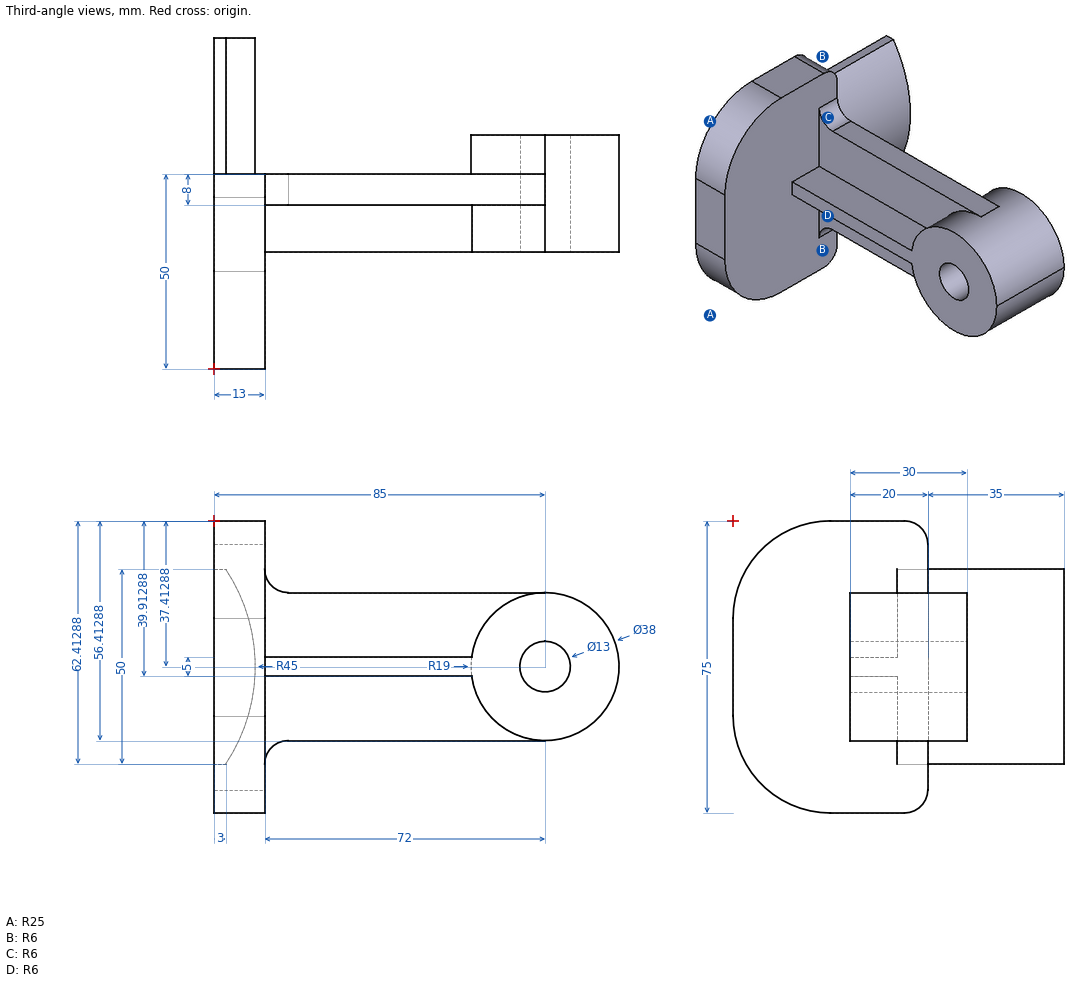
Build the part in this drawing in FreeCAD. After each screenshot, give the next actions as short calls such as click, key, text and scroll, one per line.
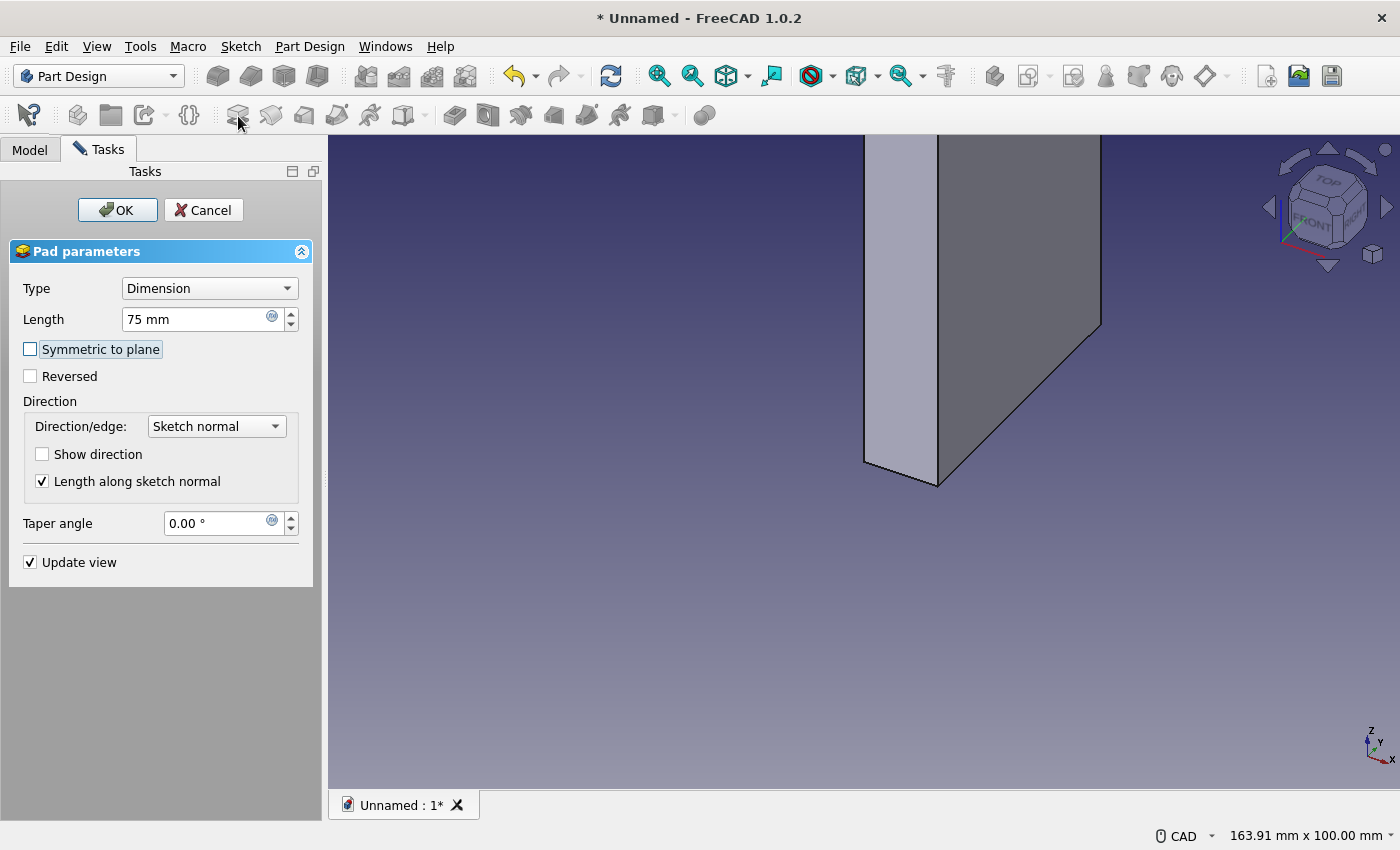
click(31, 376)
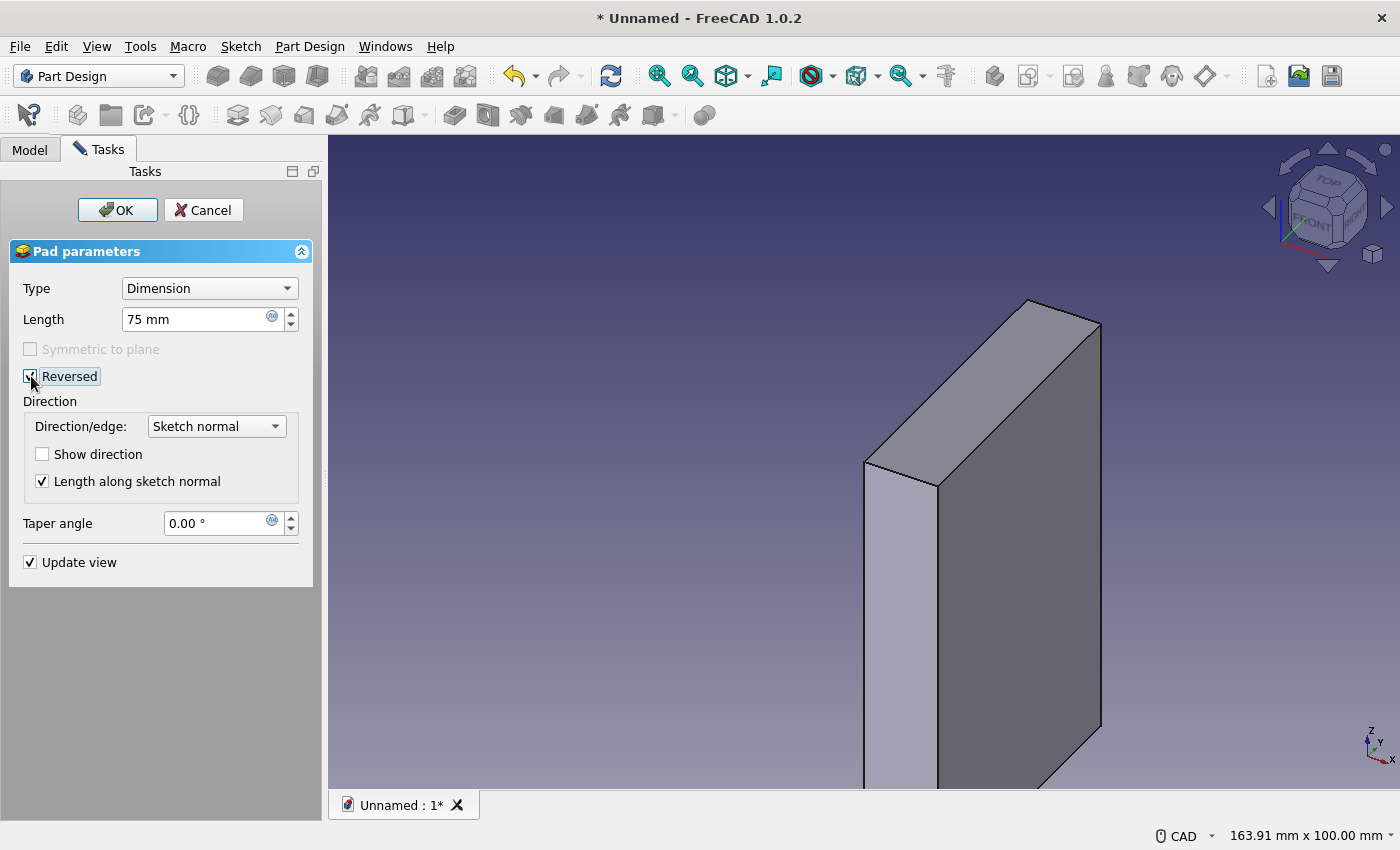
click(118, 210)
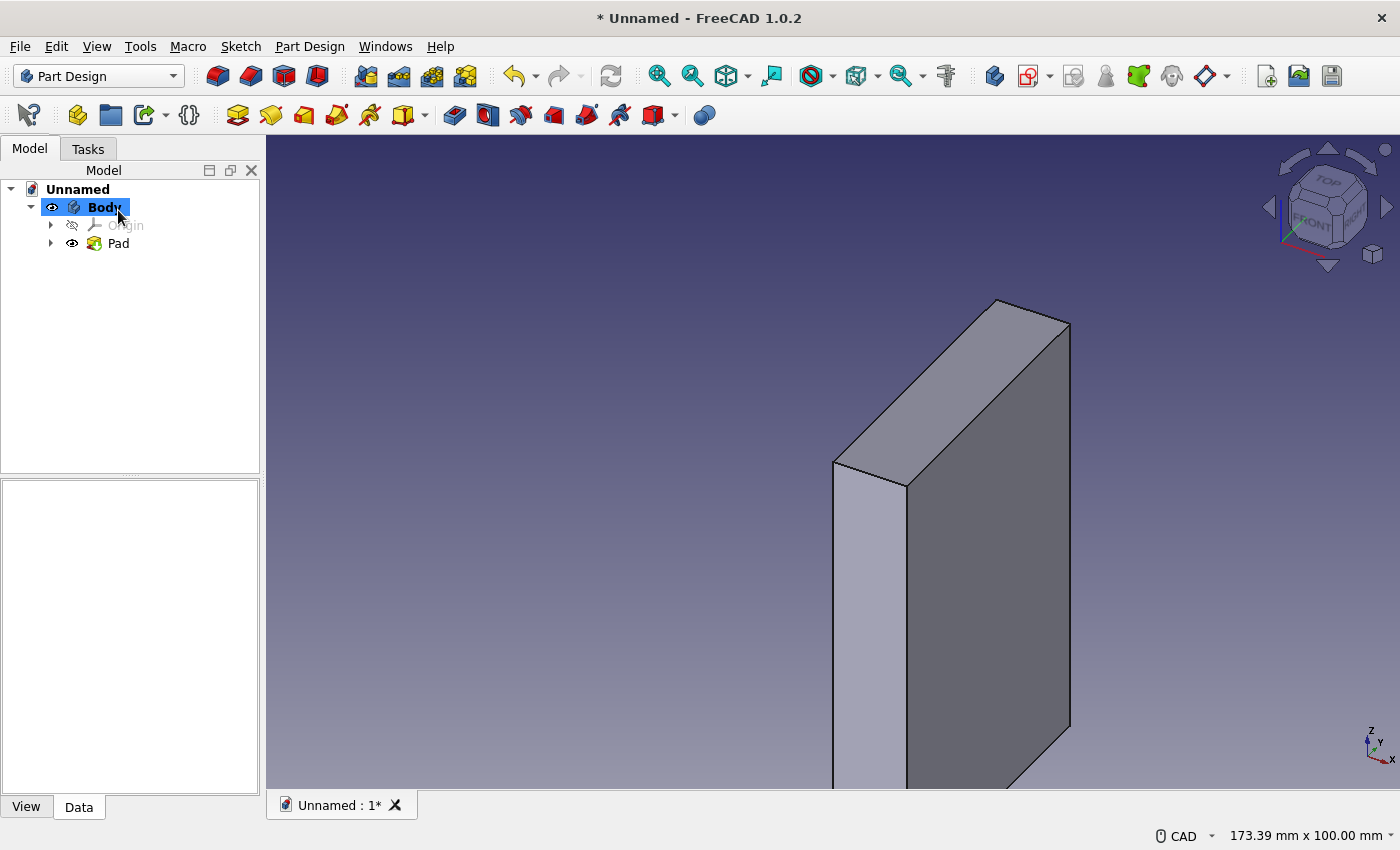
click(660, 76)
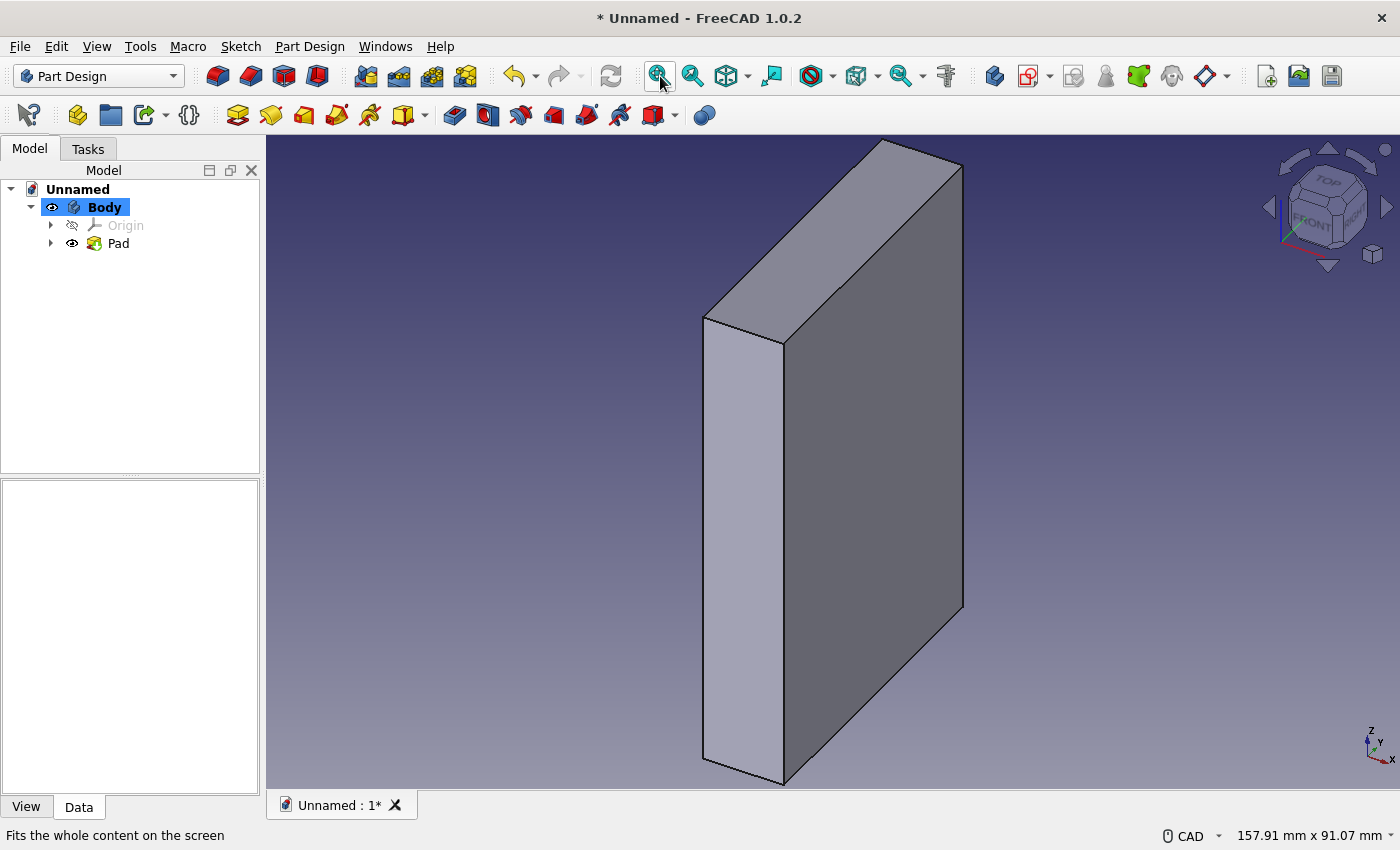
click(743, 330)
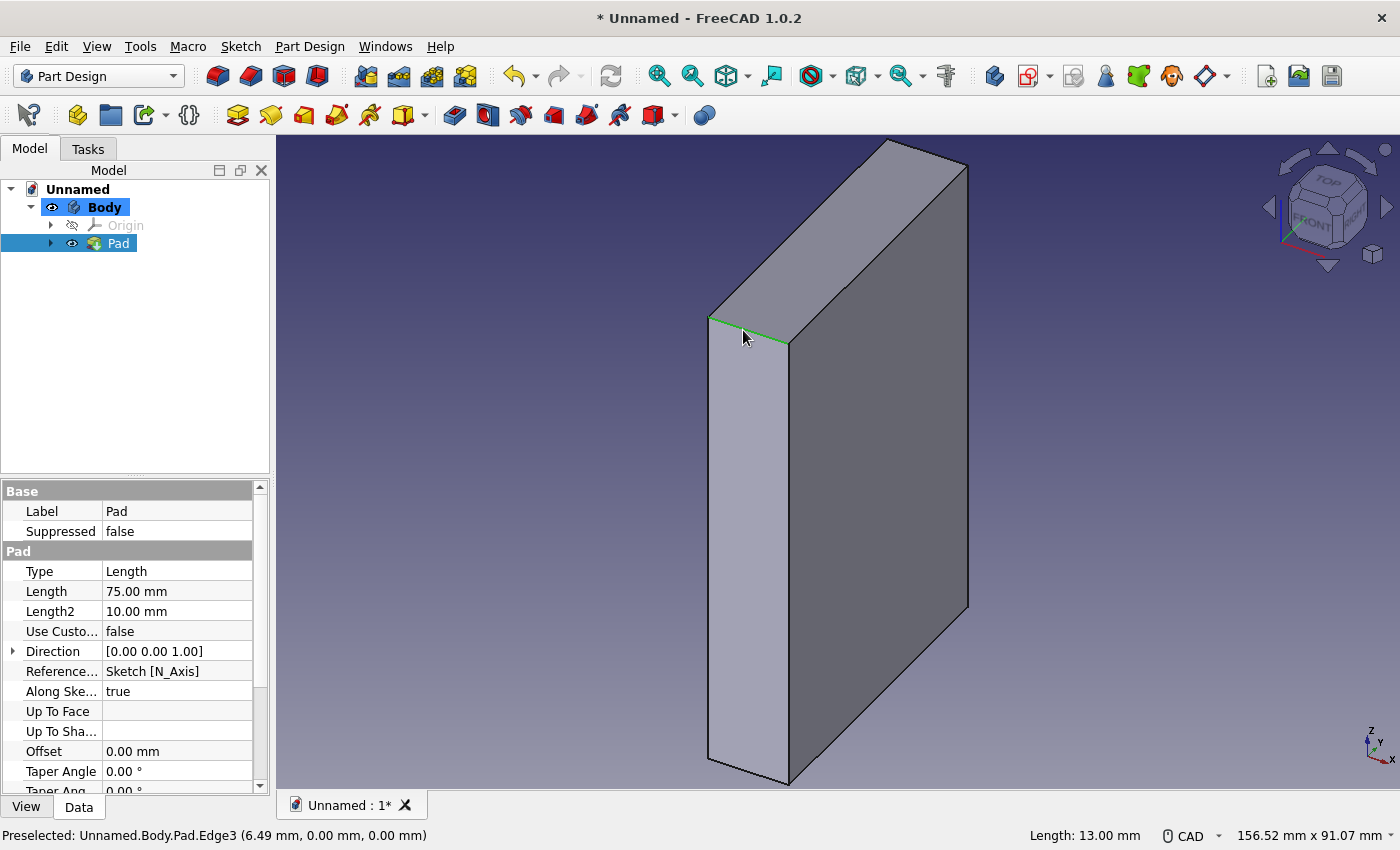
key(0)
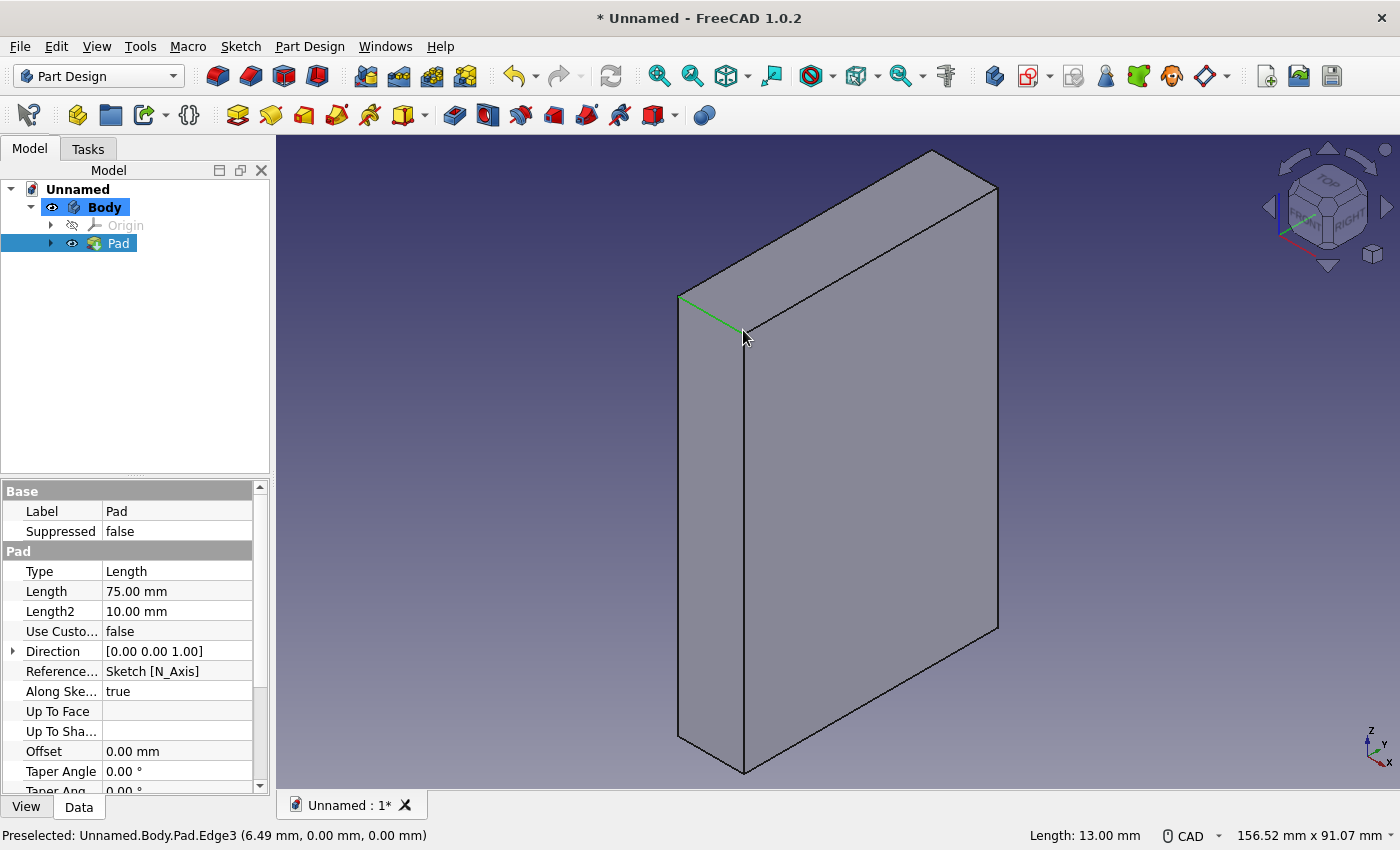
key(2)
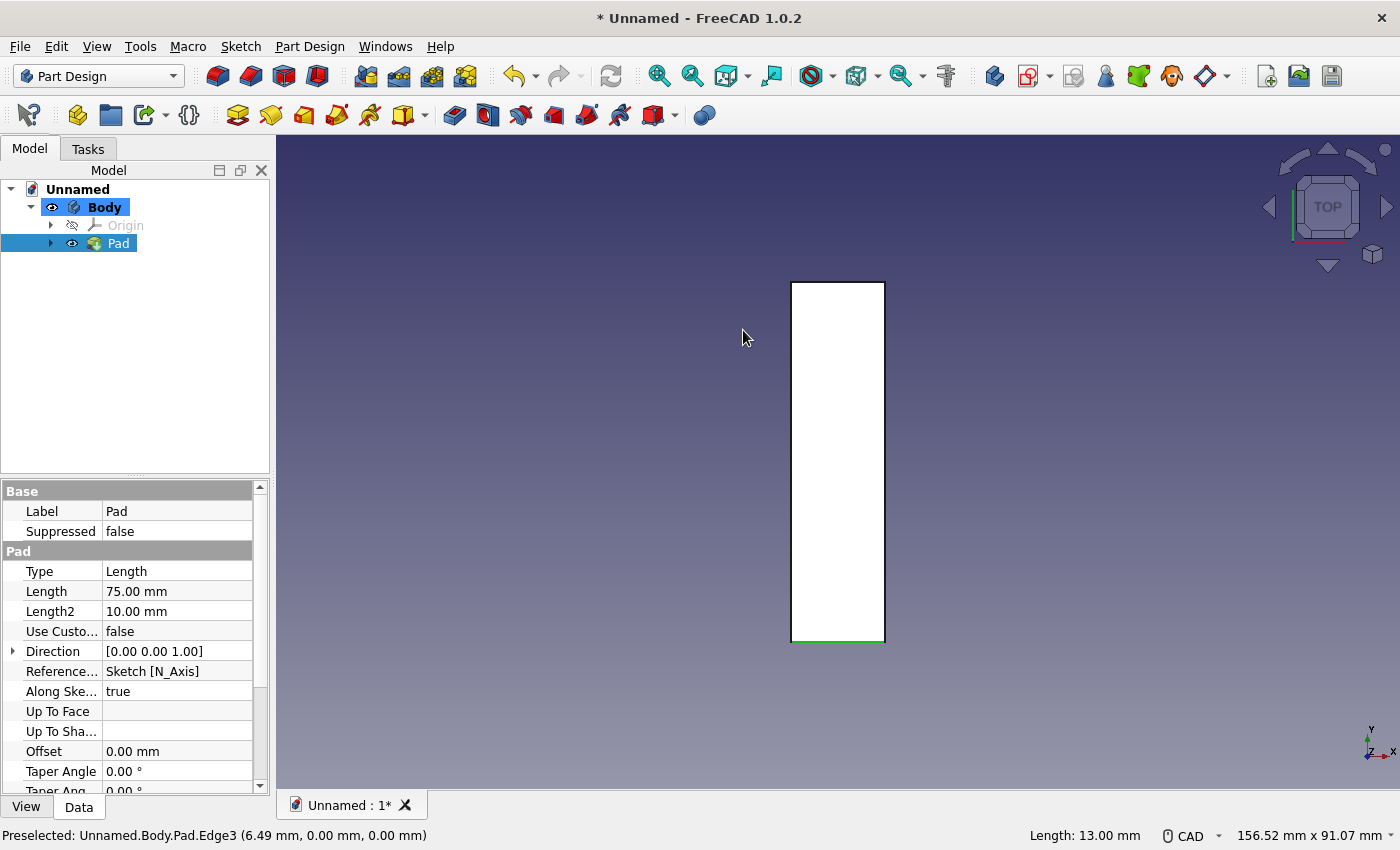
key(1)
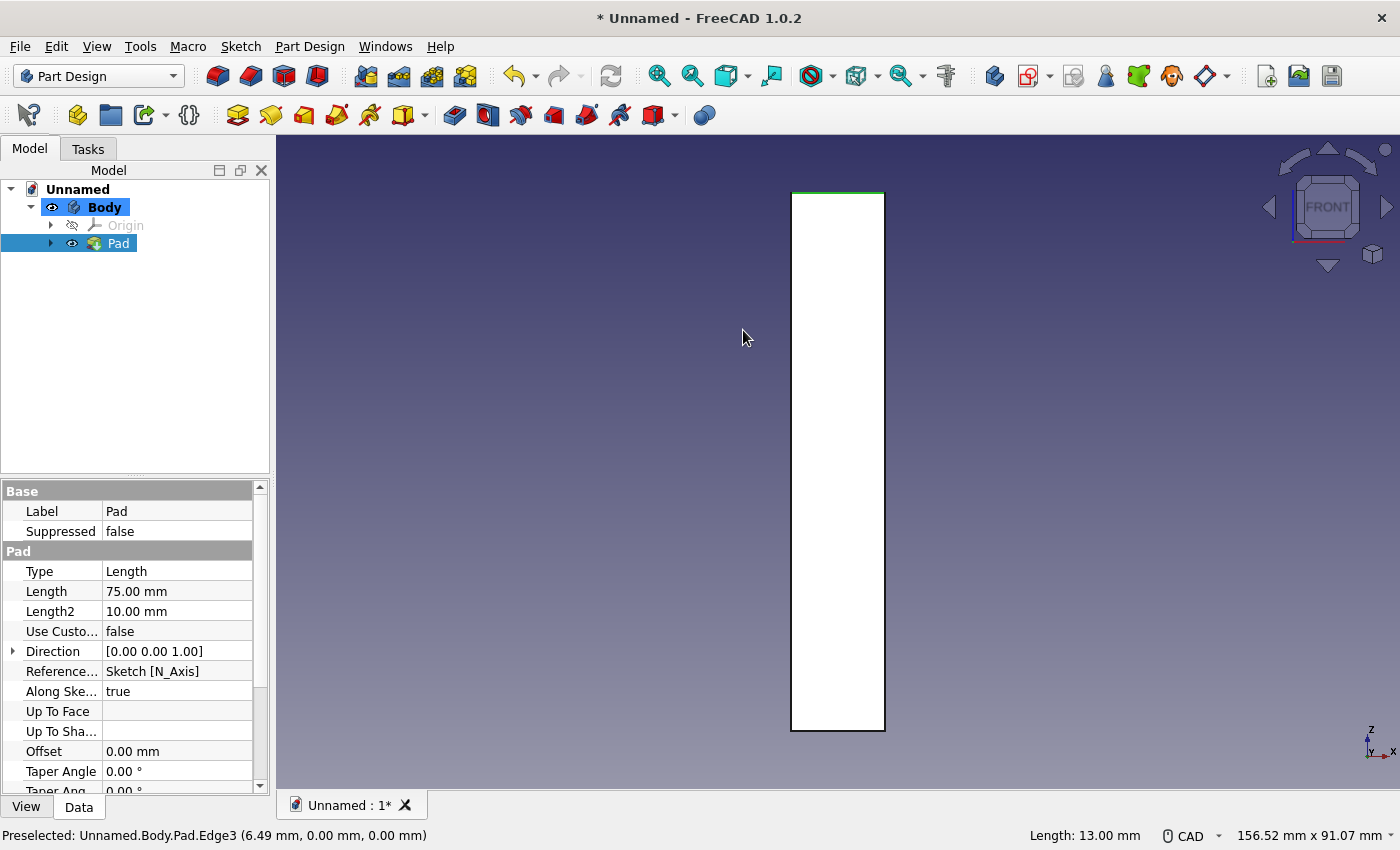
click(838, 730, ctrl)